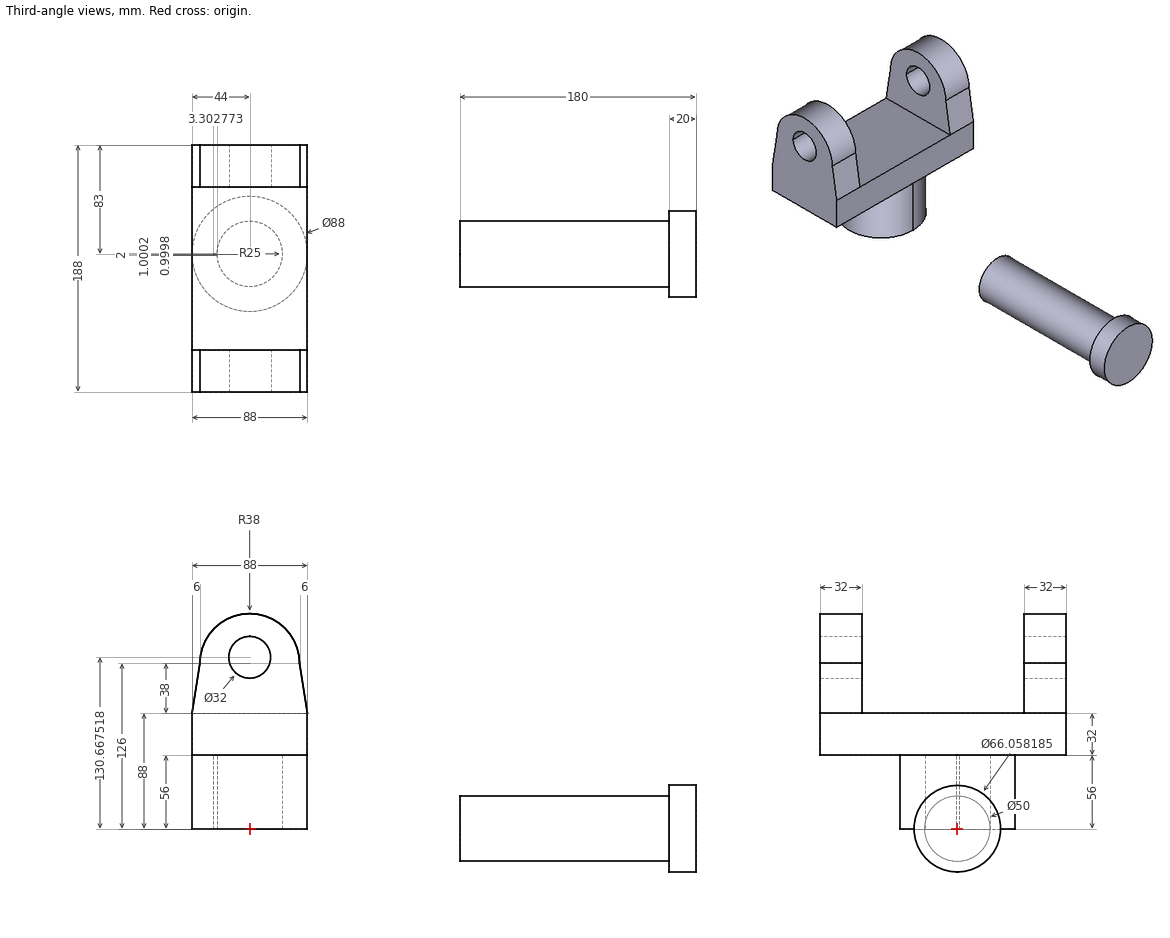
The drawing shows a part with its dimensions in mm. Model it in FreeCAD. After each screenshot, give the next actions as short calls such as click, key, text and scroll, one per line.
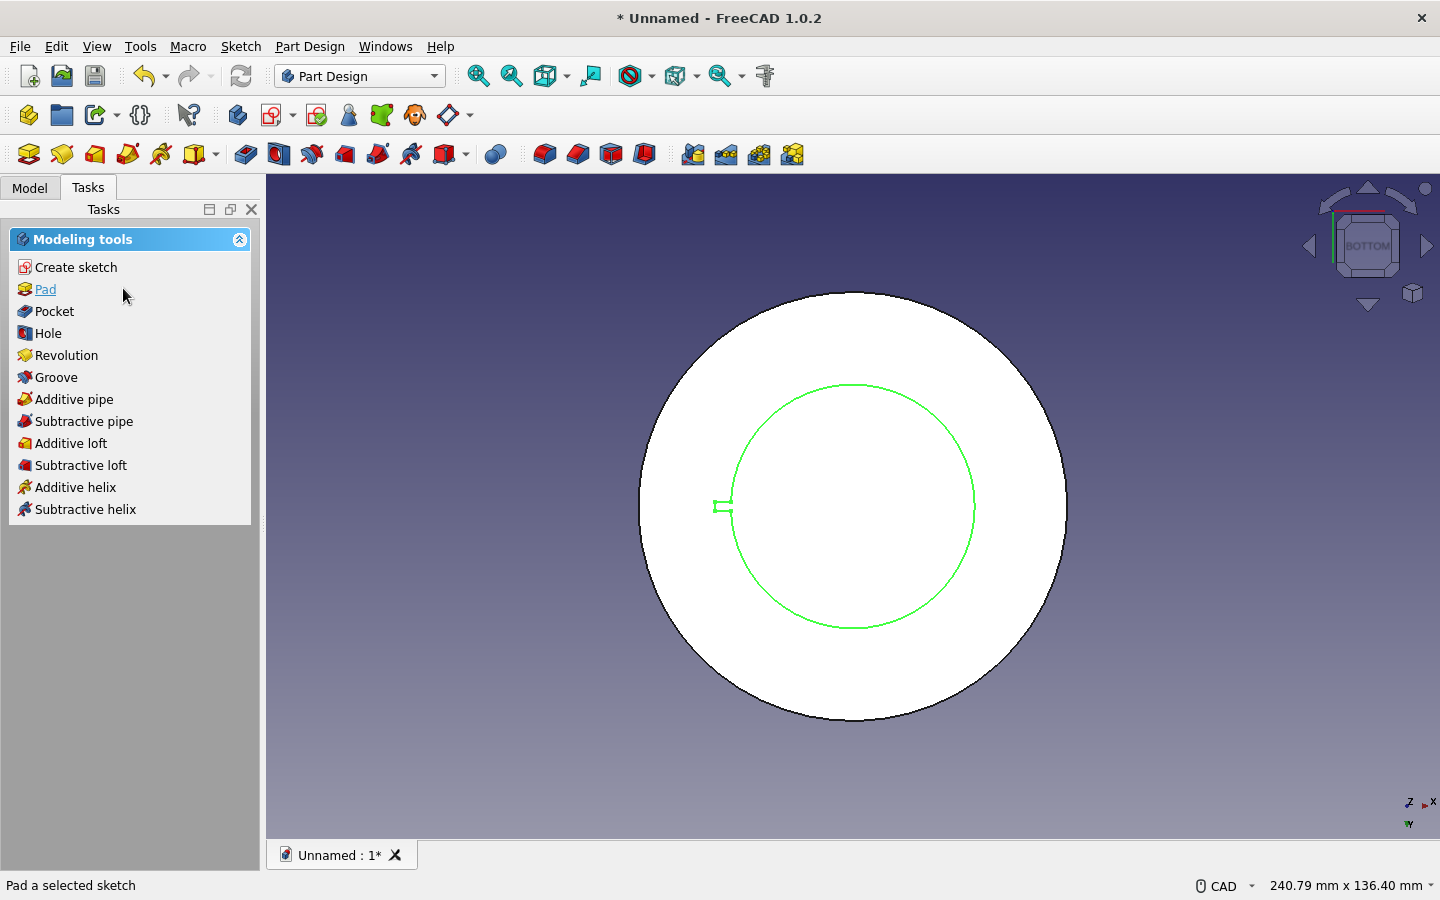
click(246, 154)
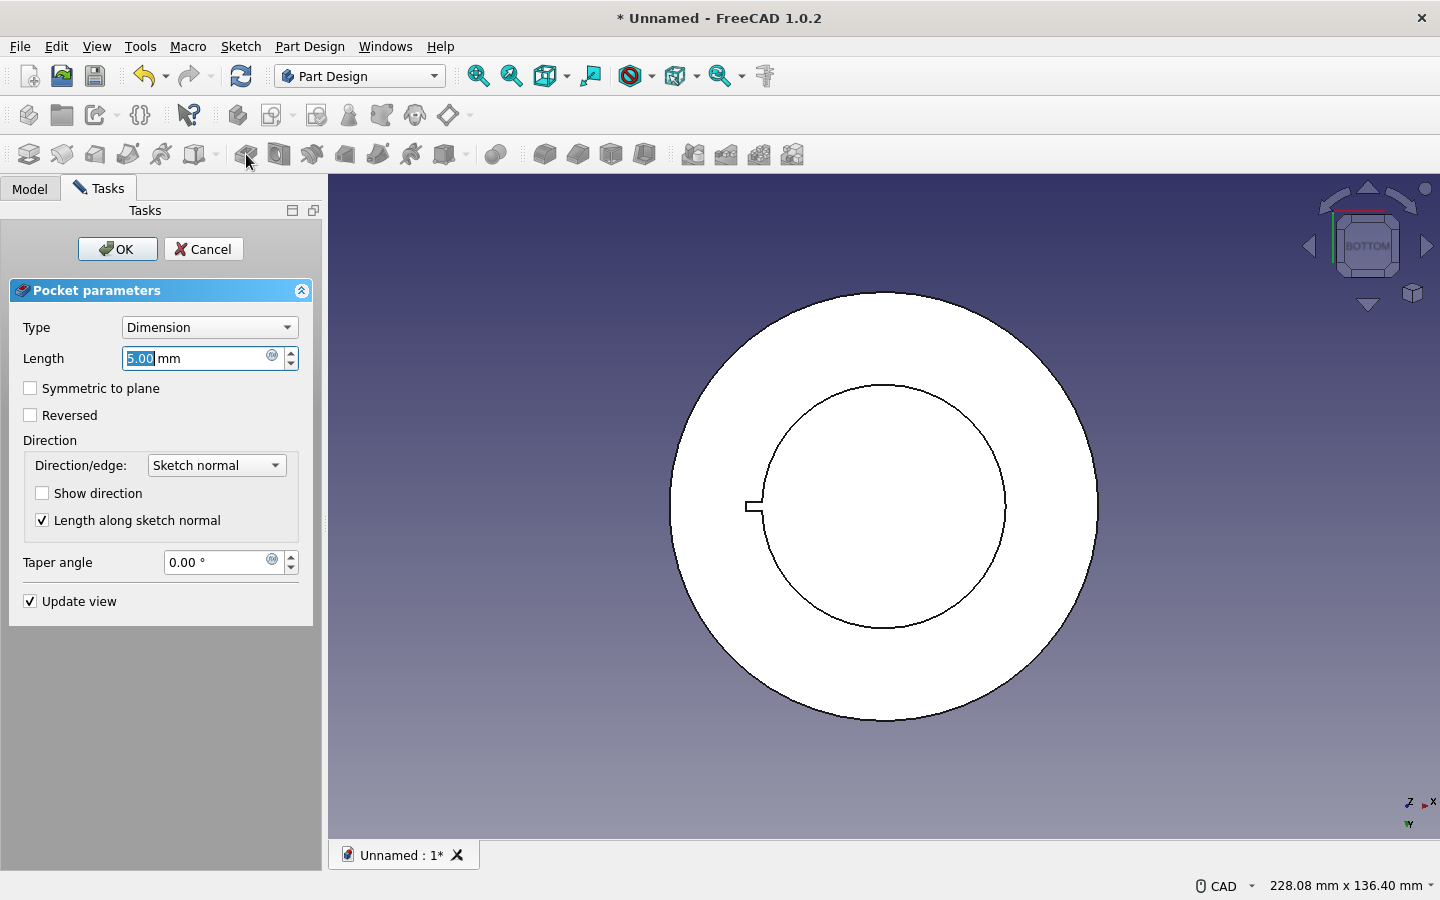
text(56)
key(Tab)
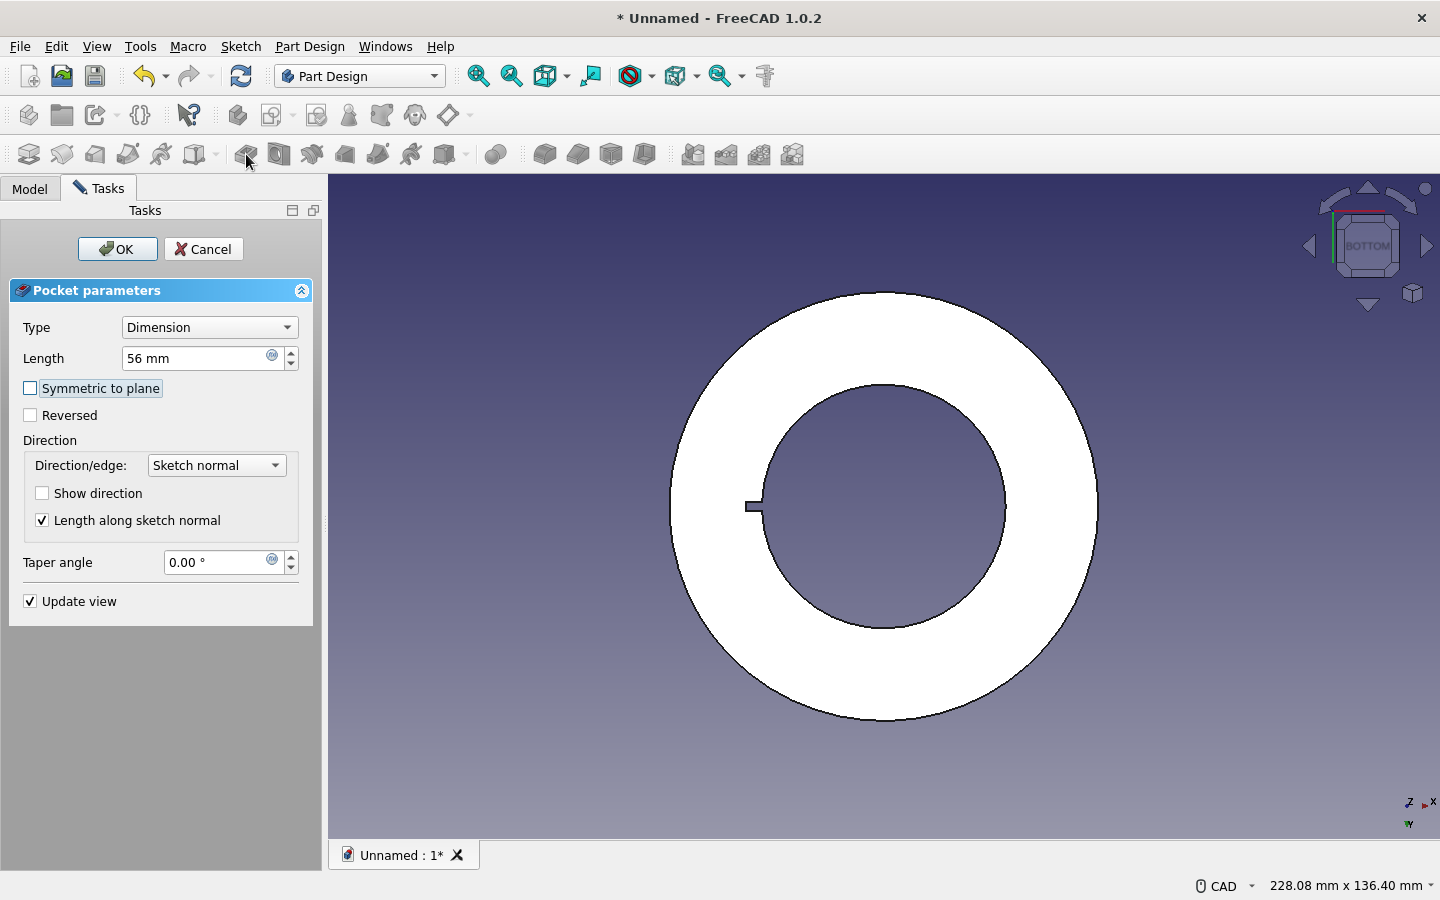
click(118, 249)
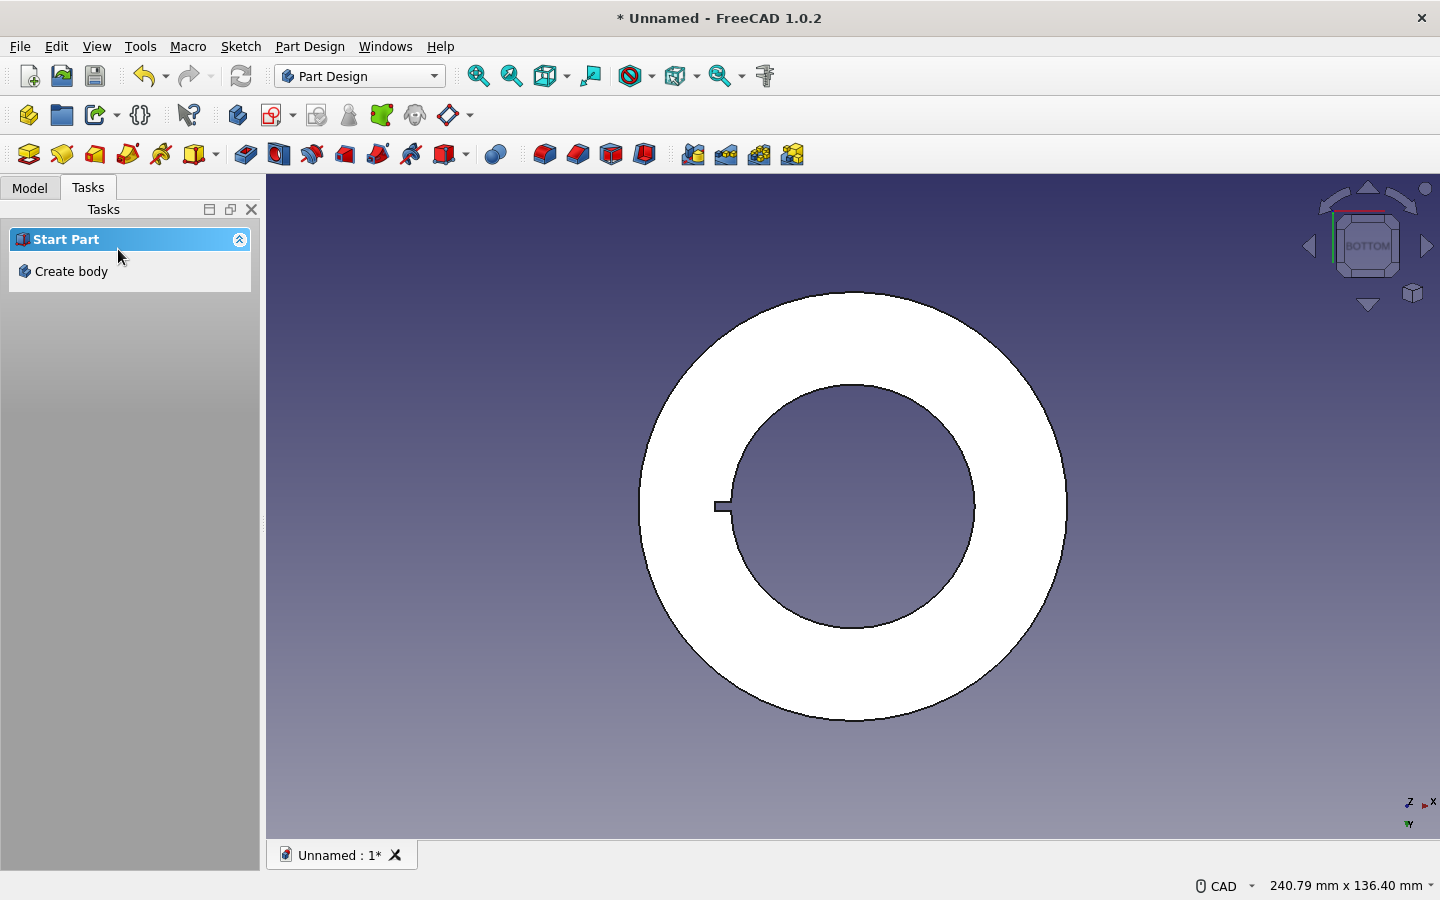
key(0)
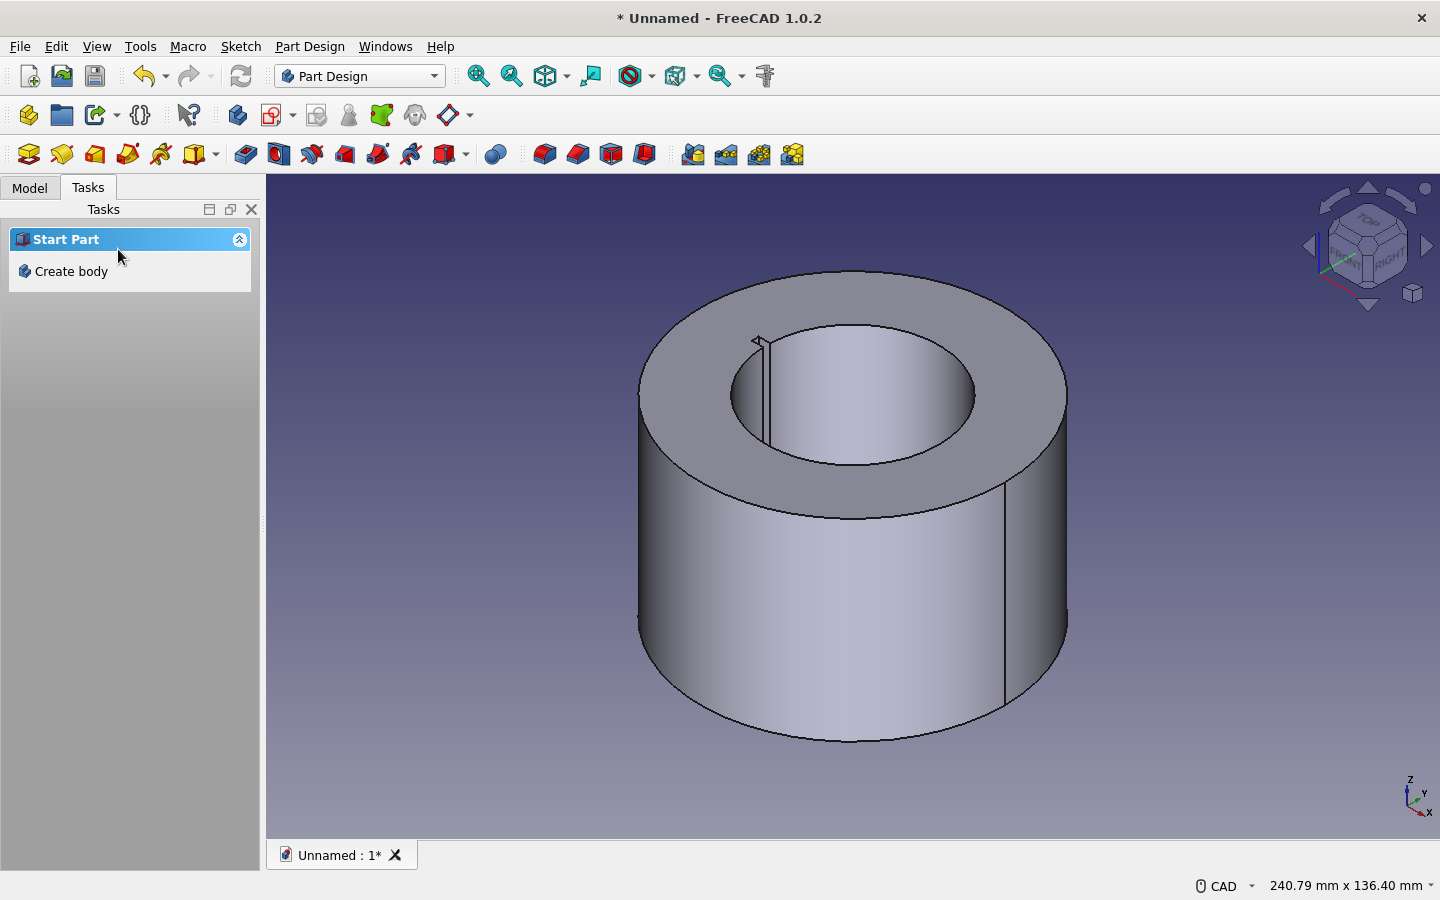
click(1026, 394)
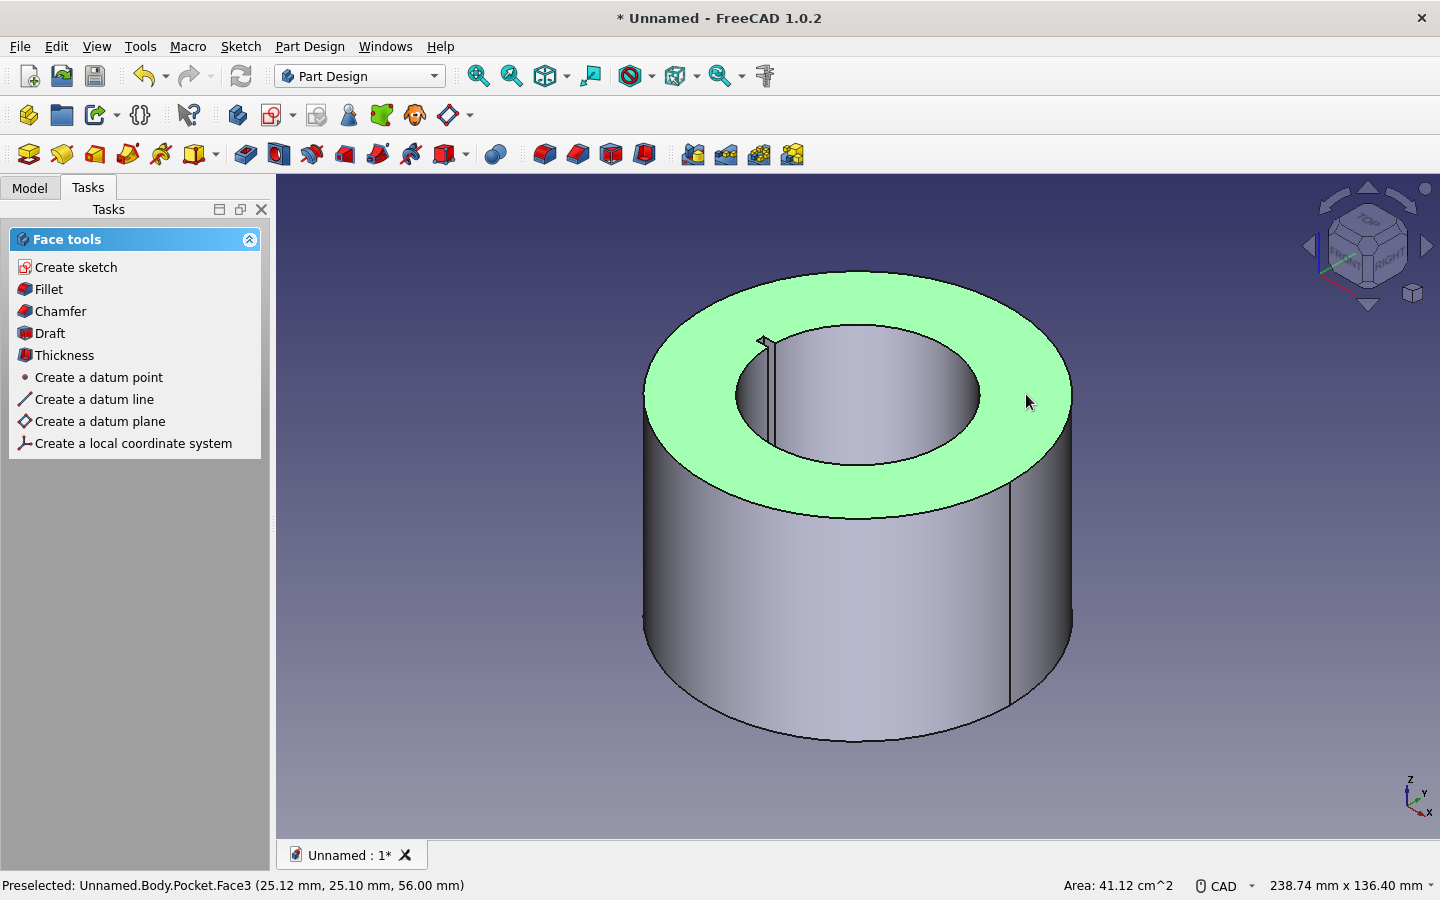
click(270, 116)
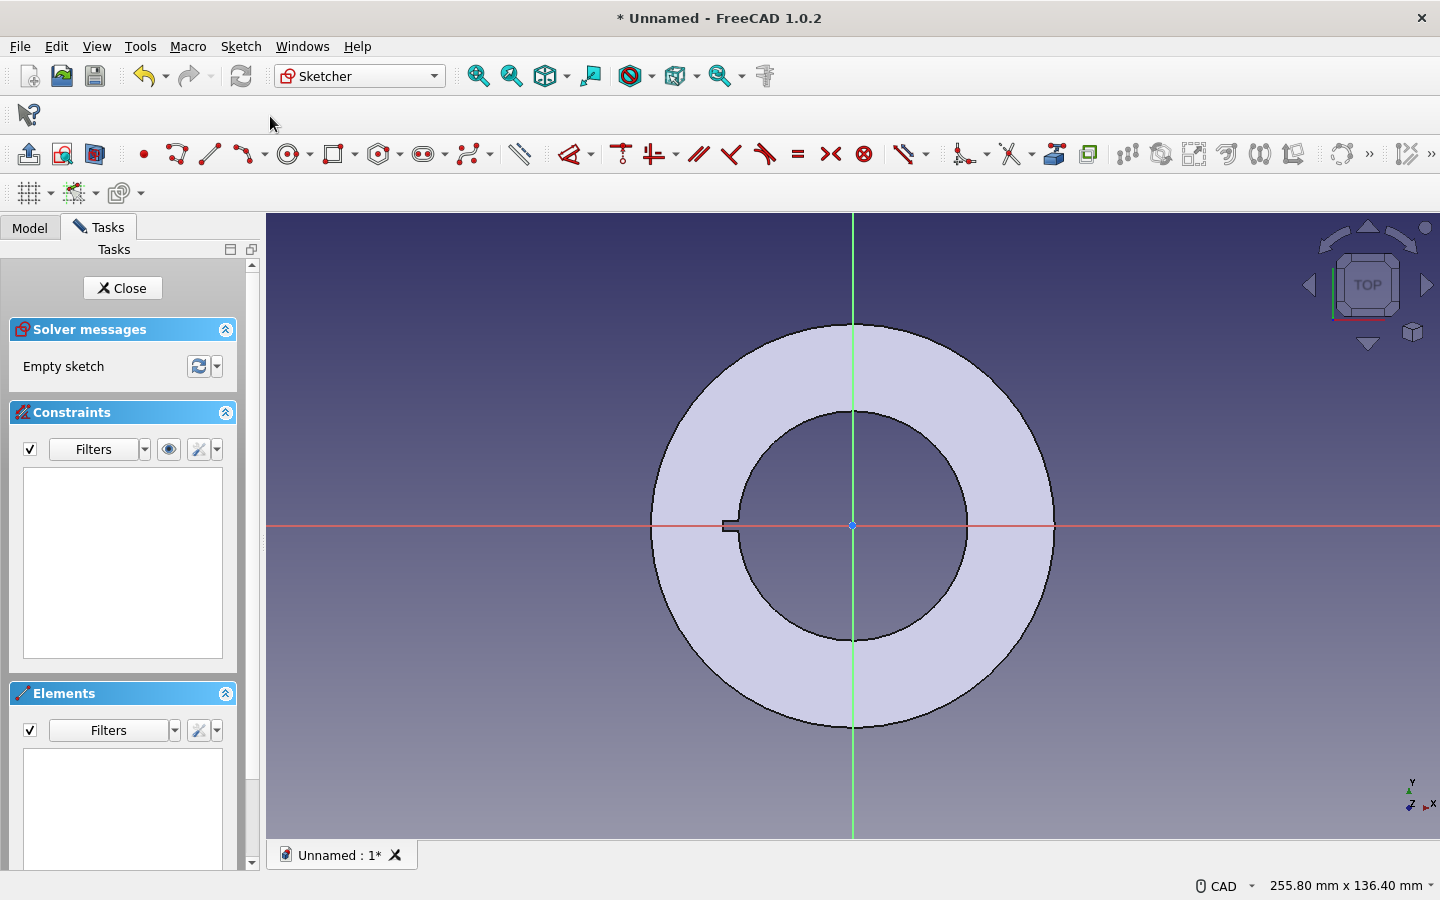
scroll(729, 485, down, 4)